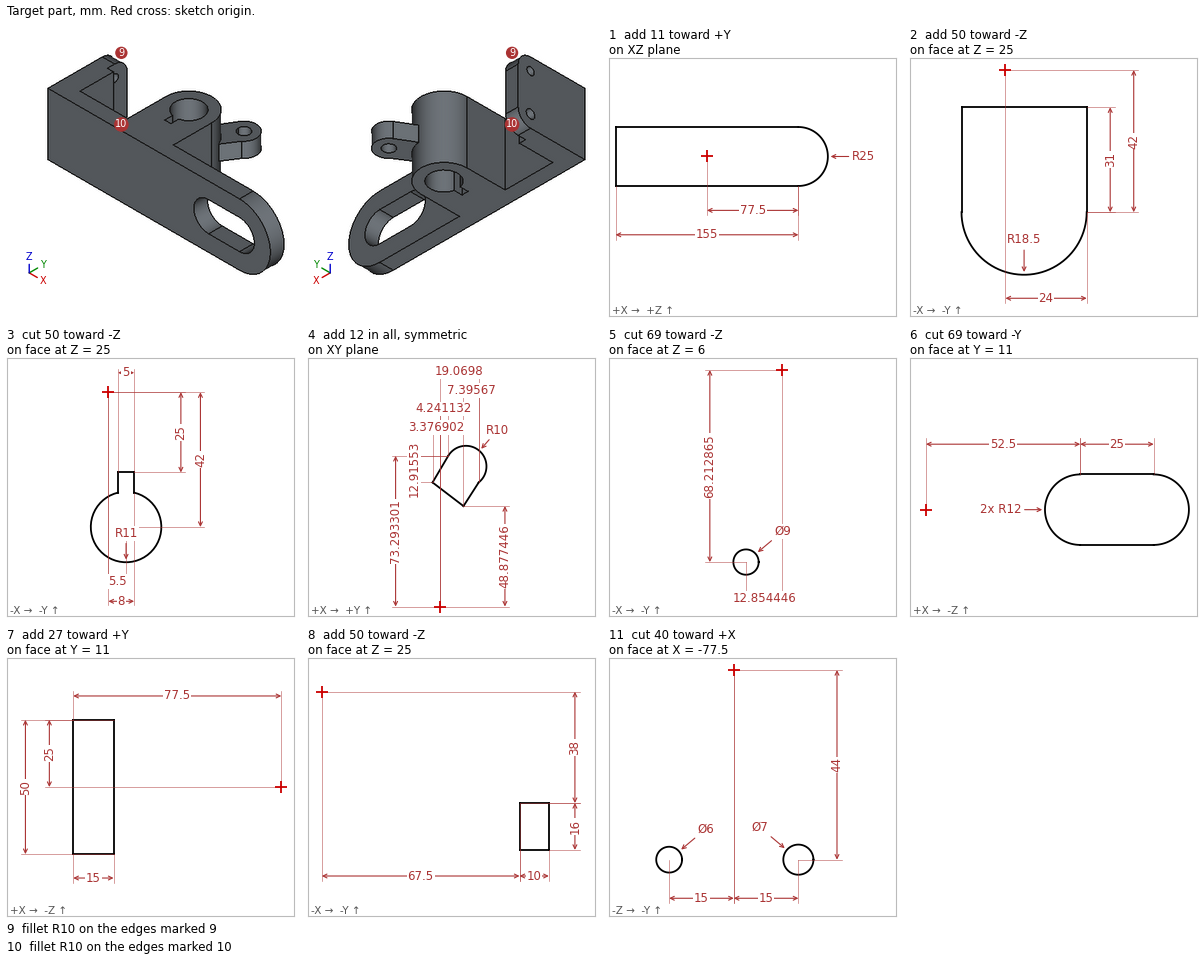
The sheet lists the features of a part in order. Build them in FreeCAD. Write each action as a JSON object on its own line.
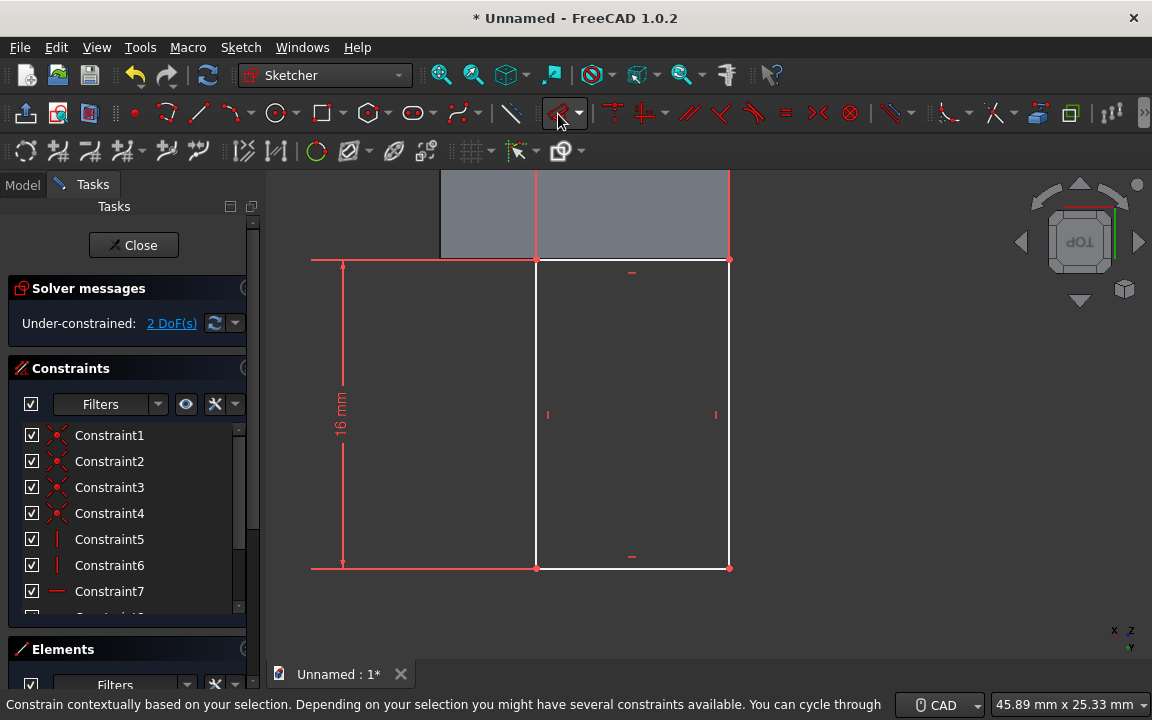
{"action": "left_click", "coordinate": [536, 260]}
{"action": "left_click", "coordinate": [570, 229]}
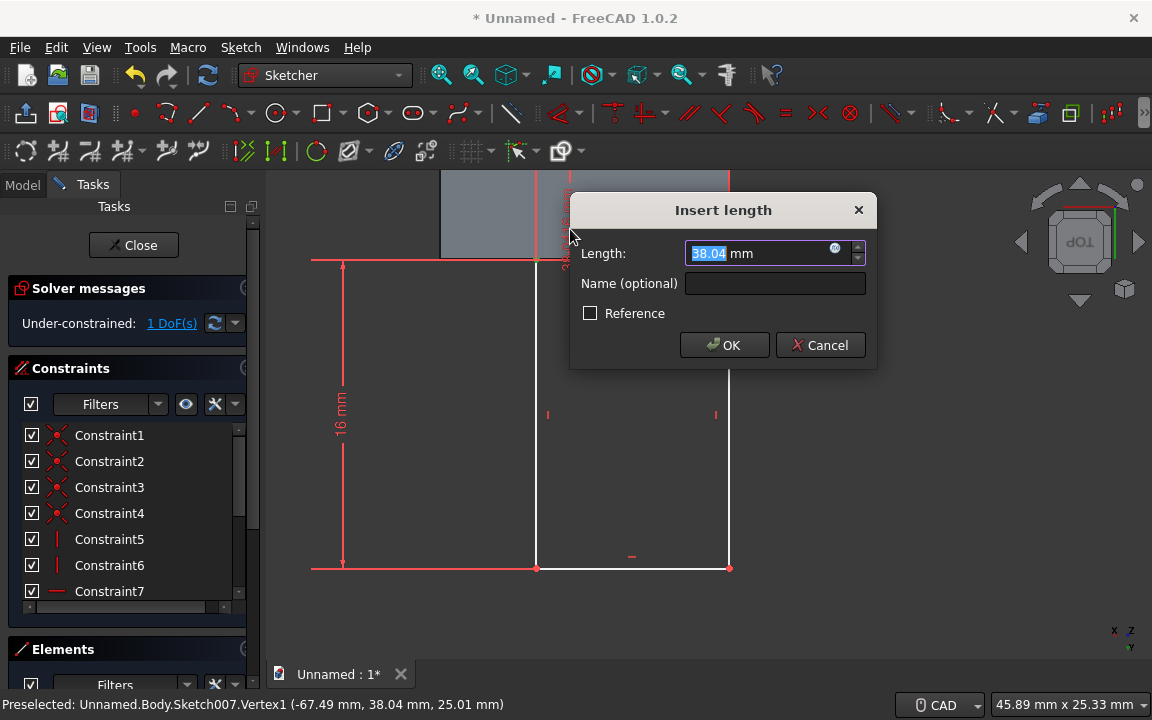
{"action": "type", "text": "38"}
{"action": "key", "text": "Return"}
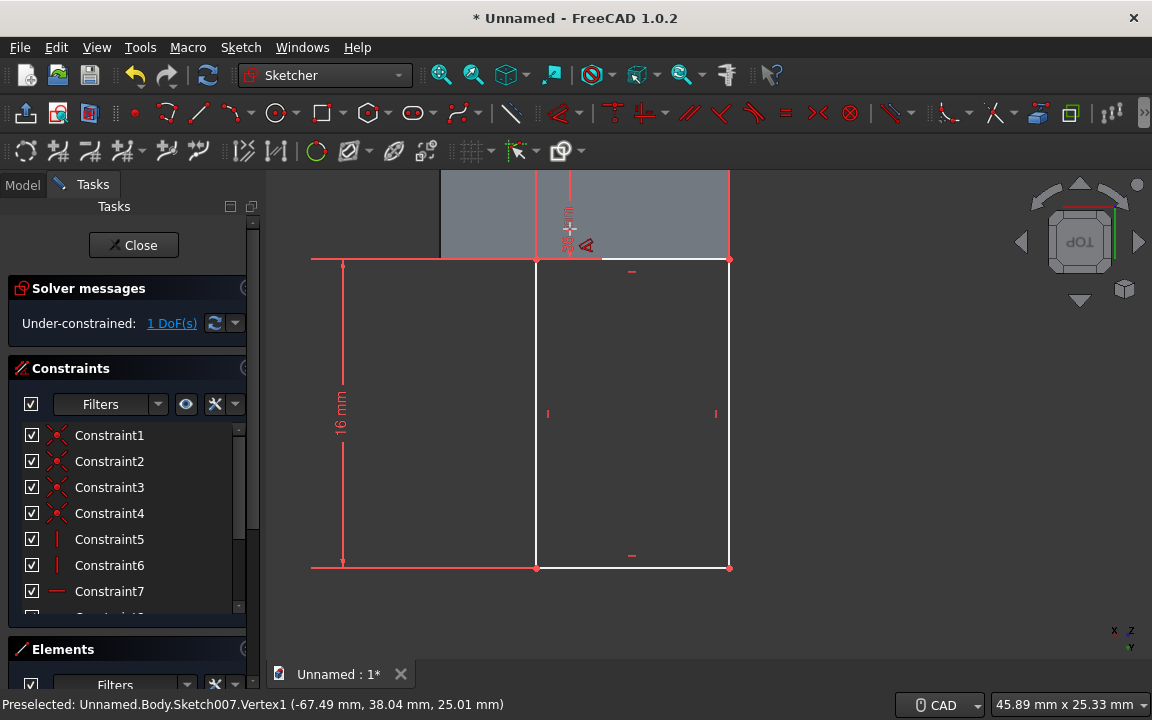
{"action": "left_click", "coordinate": [536, 259]}
{"action": "left_click", "coordinate": [415, 293]}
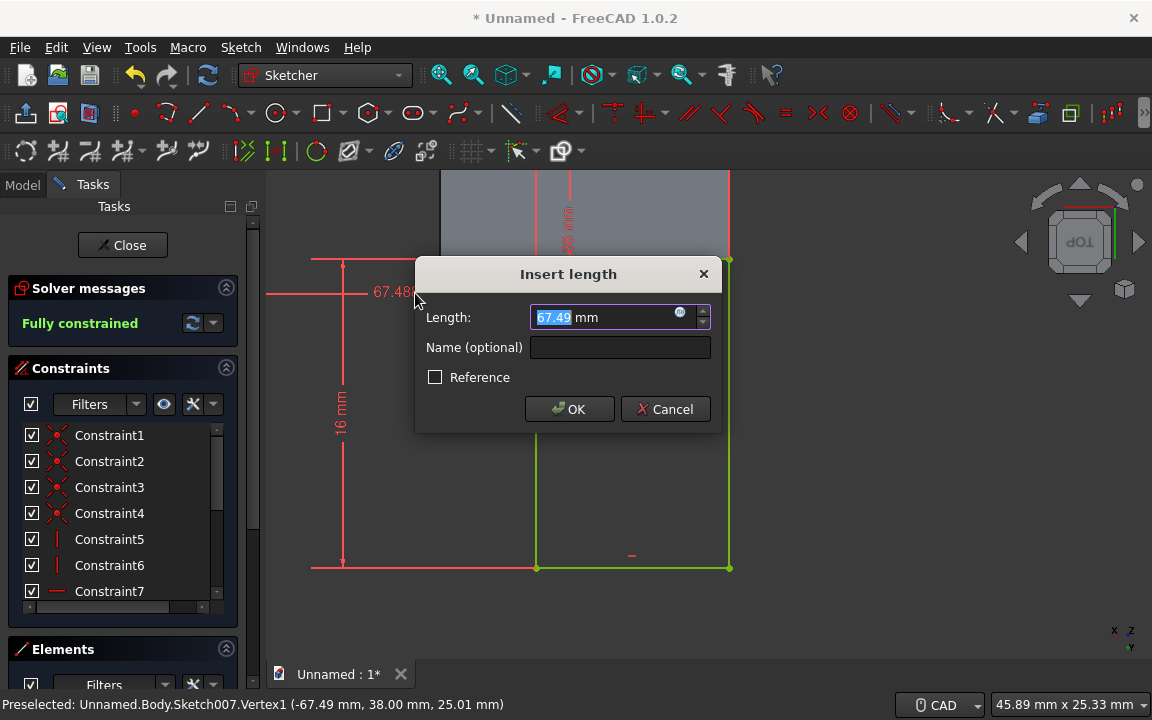
{"action": "type", "text": "67.5"}
{"action": "key", "text": "Return"}
{"action": "key", "text": "Escape"}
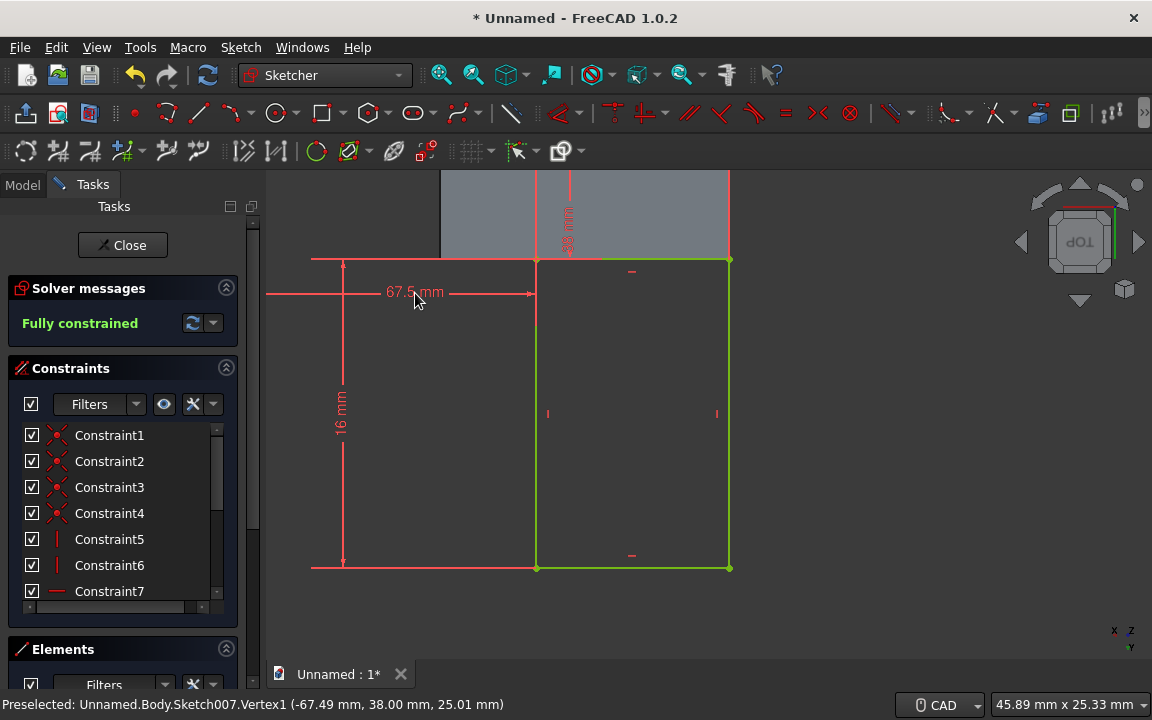
{"action": "left_click", "coordinate": [123, 245]}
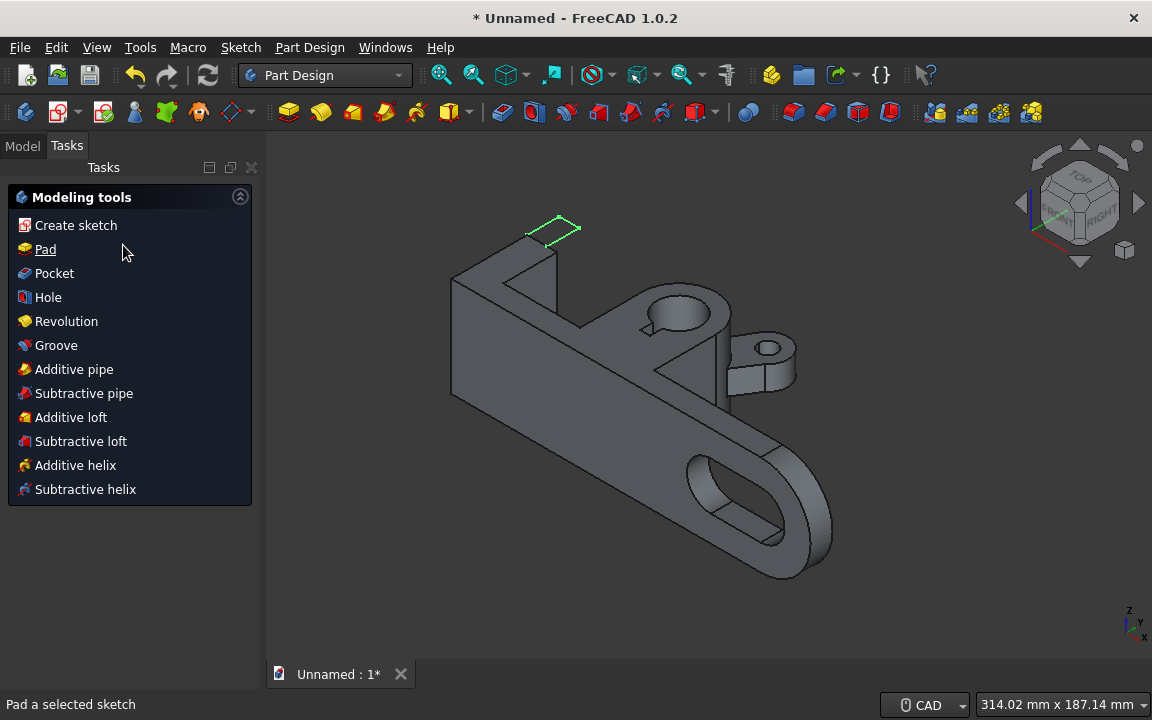
{"action": "left_click", "coordinate": [290, 112]}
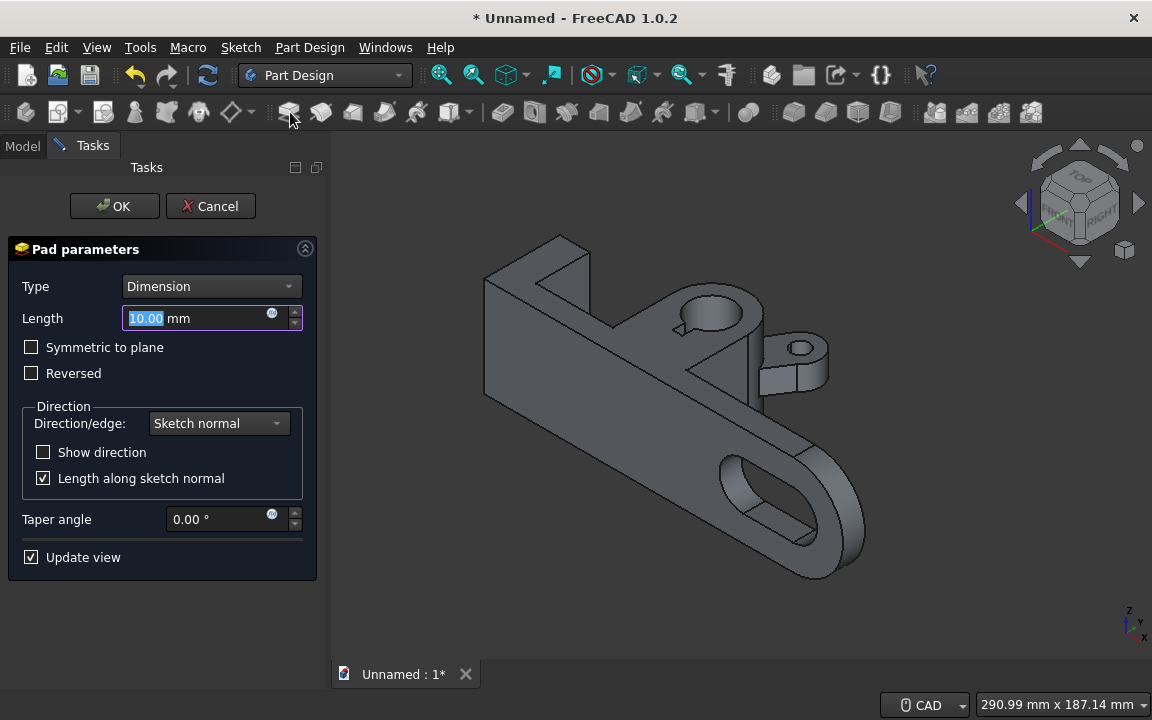
{"action": "type", "text": "50"}
{"action": "key", "text": "Tab"}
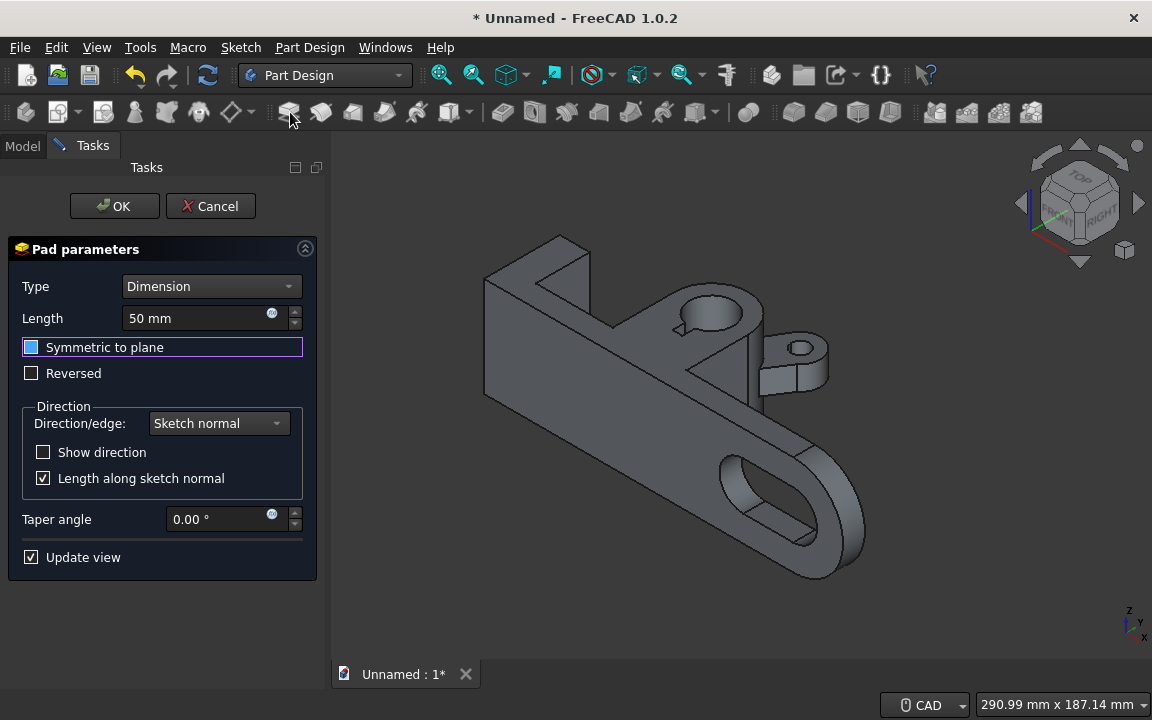
{"action": "left_click", "coordinate": [30, 373]}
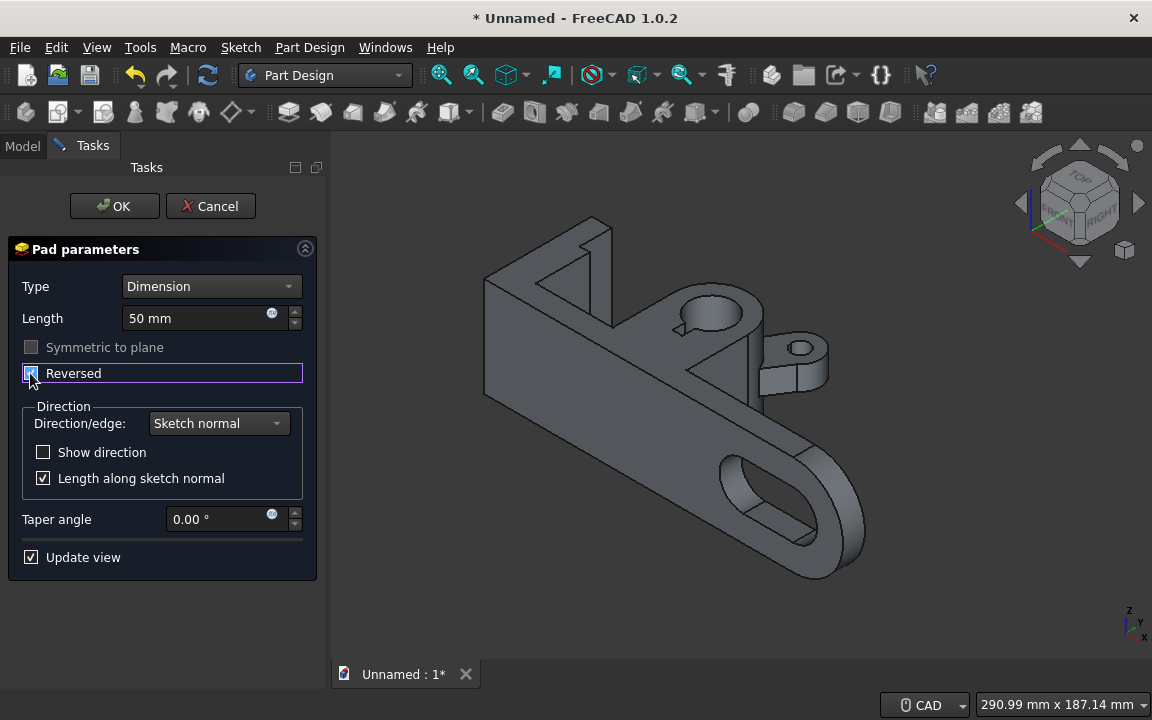
{"action": "left_click", "coordinate": [115, 206]}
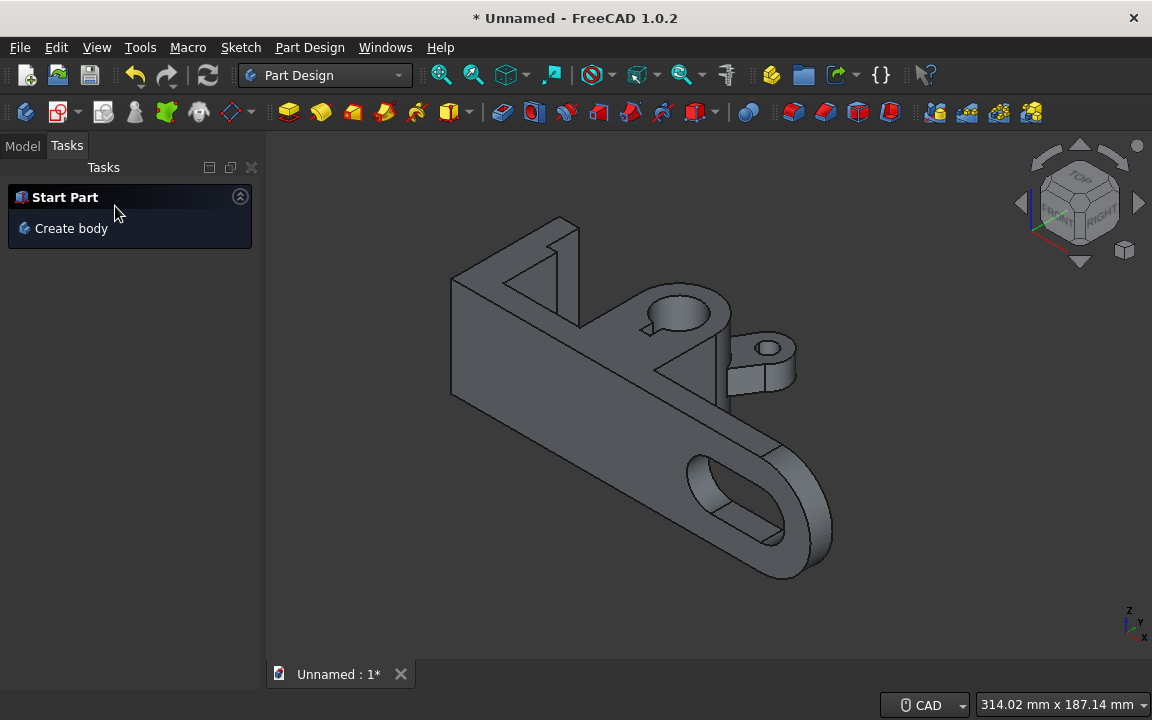
{"action": "key", "text": "2"}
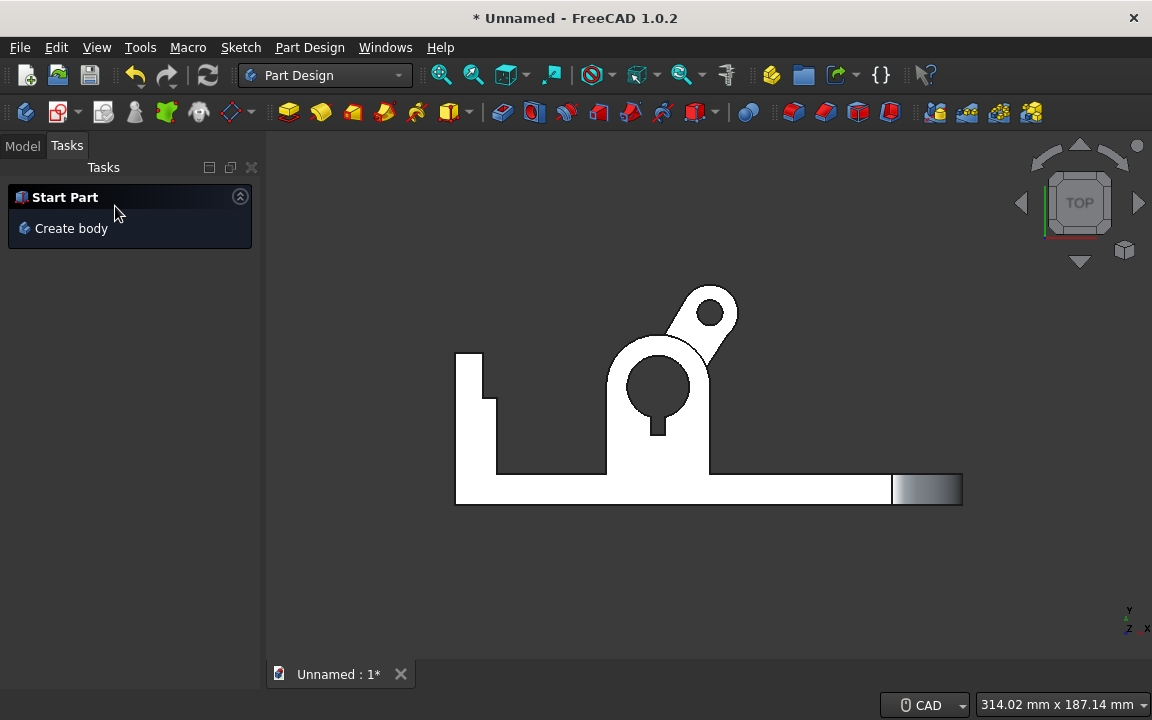
{"action": "left_click", "coordinate": [469, 352]}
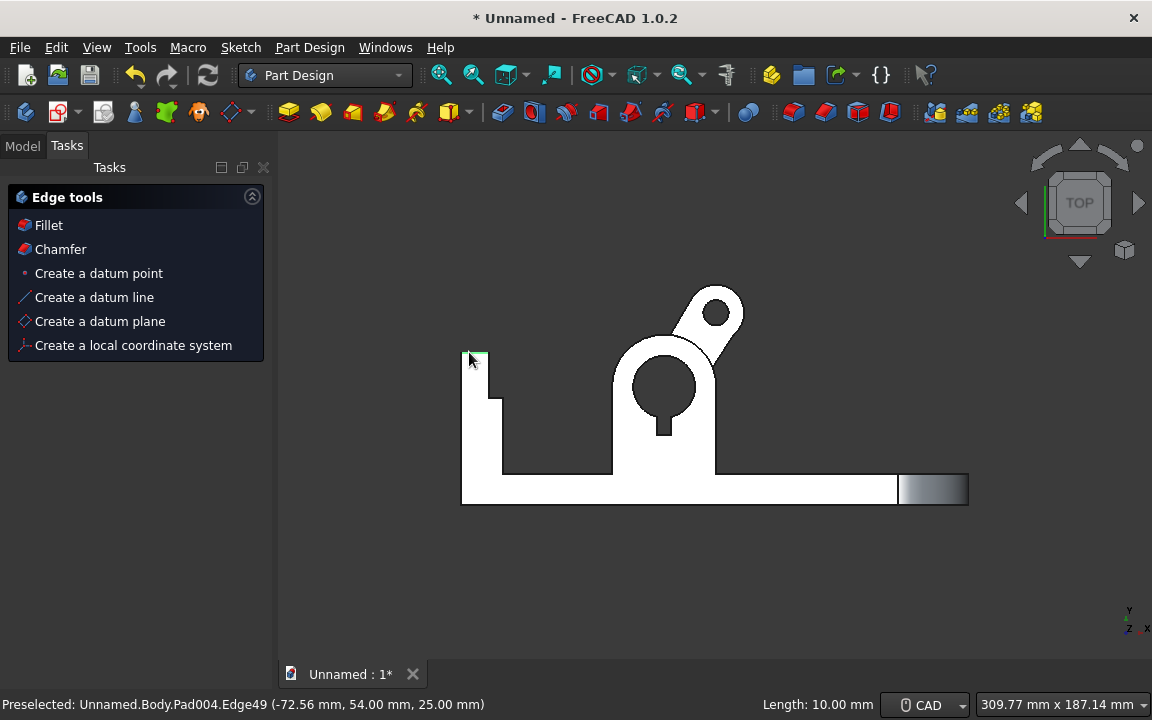
{"action": "left_click", "coordinate": [794, 112]}